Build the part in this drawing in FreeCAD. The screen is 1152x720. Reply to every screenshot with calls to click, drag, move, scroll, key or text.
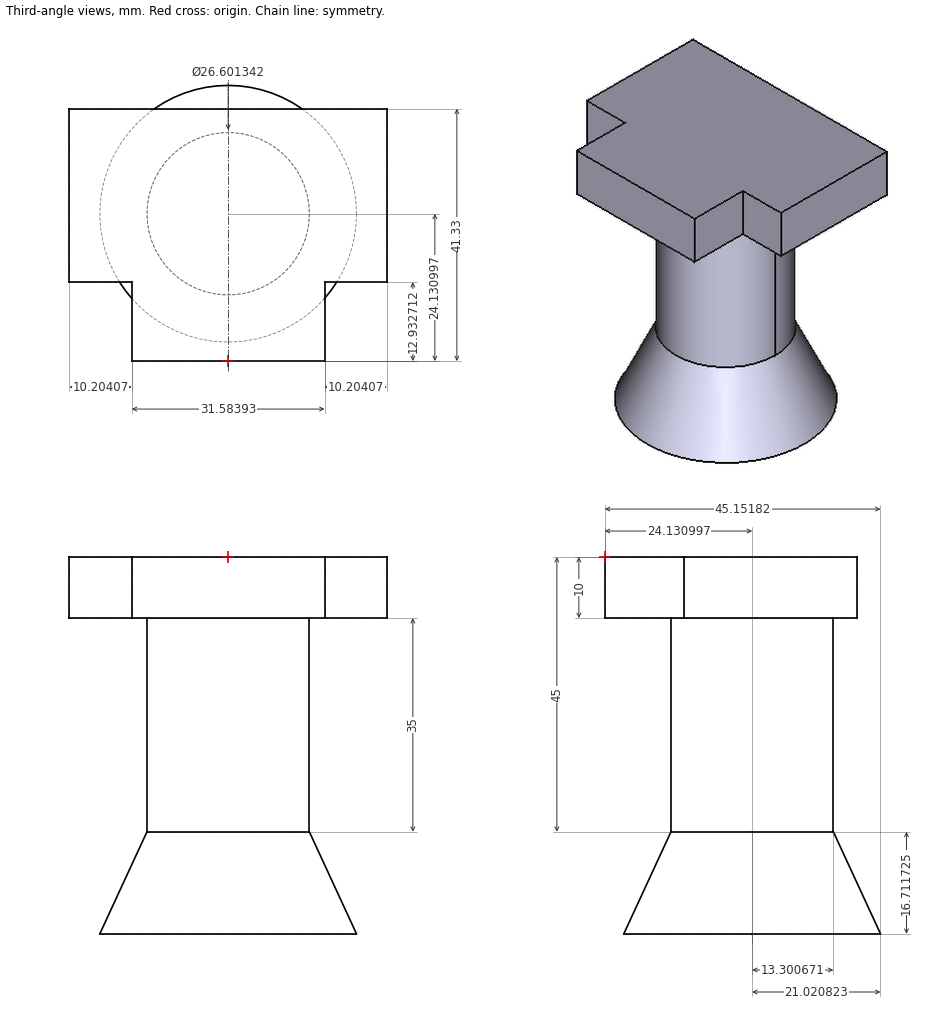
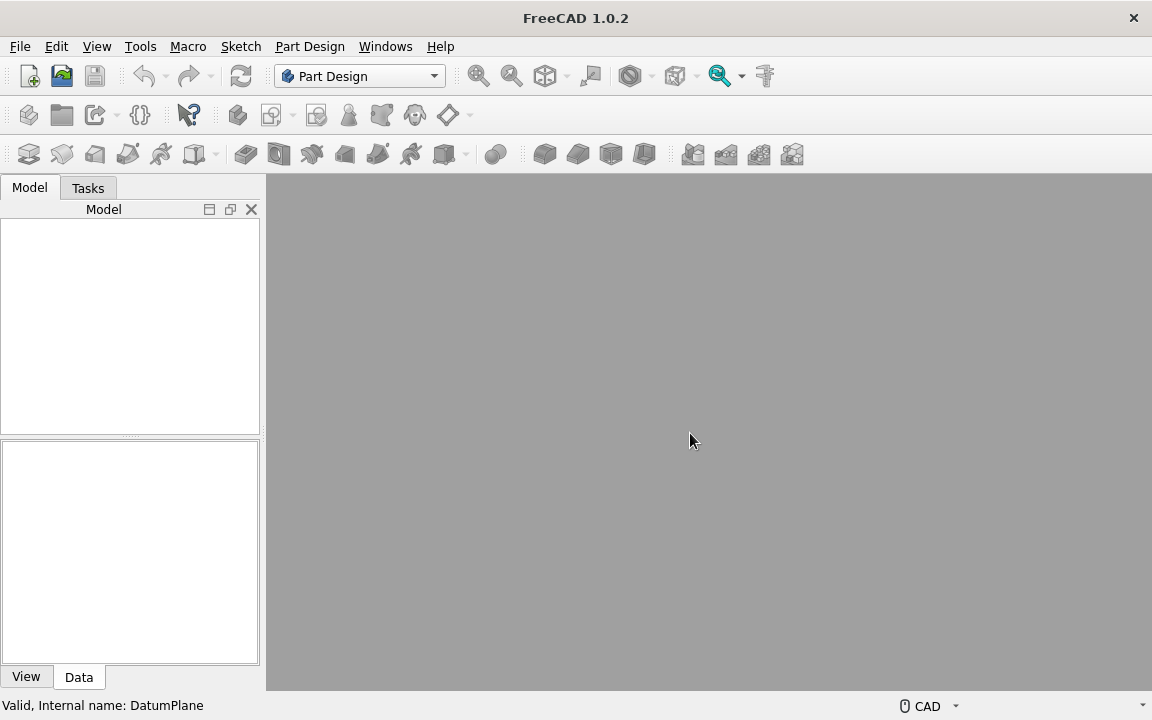
key(ctrl+n)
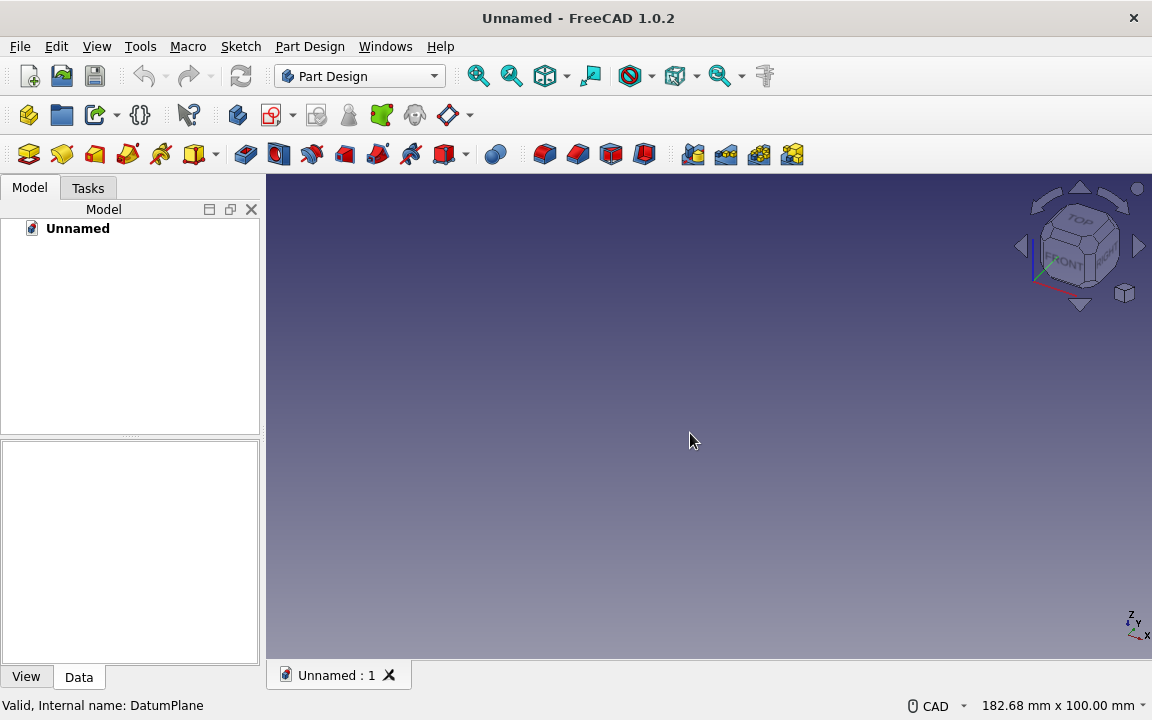
click(270, 116)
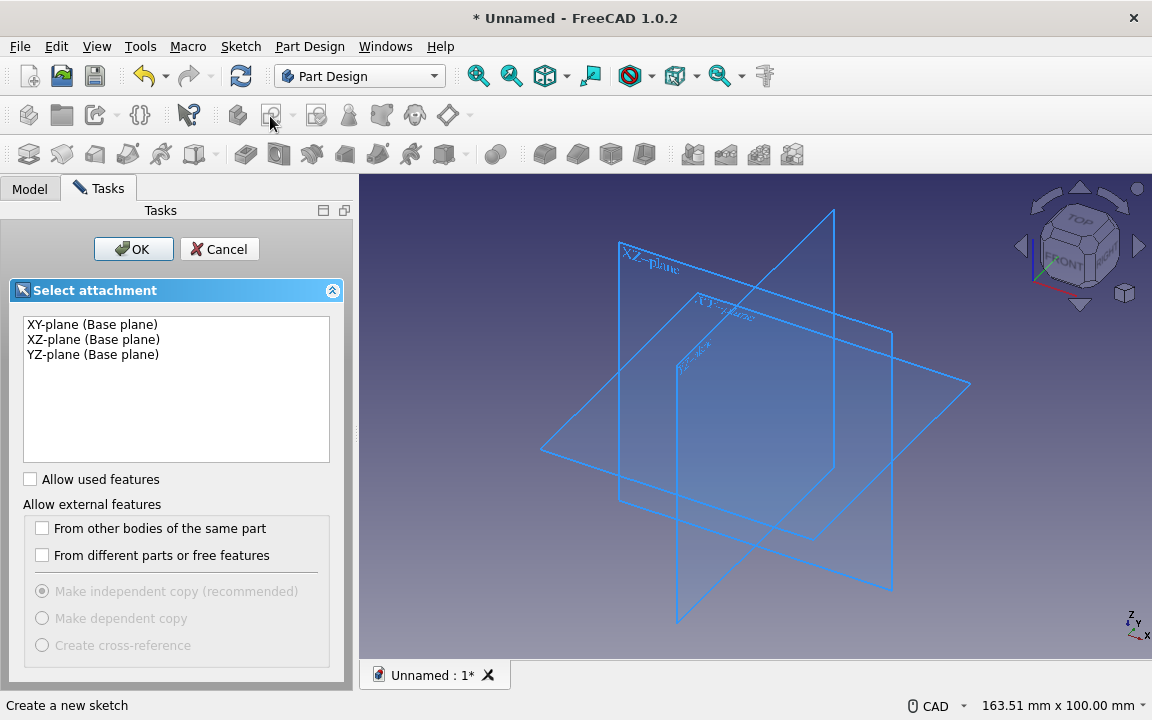
click(84, 324)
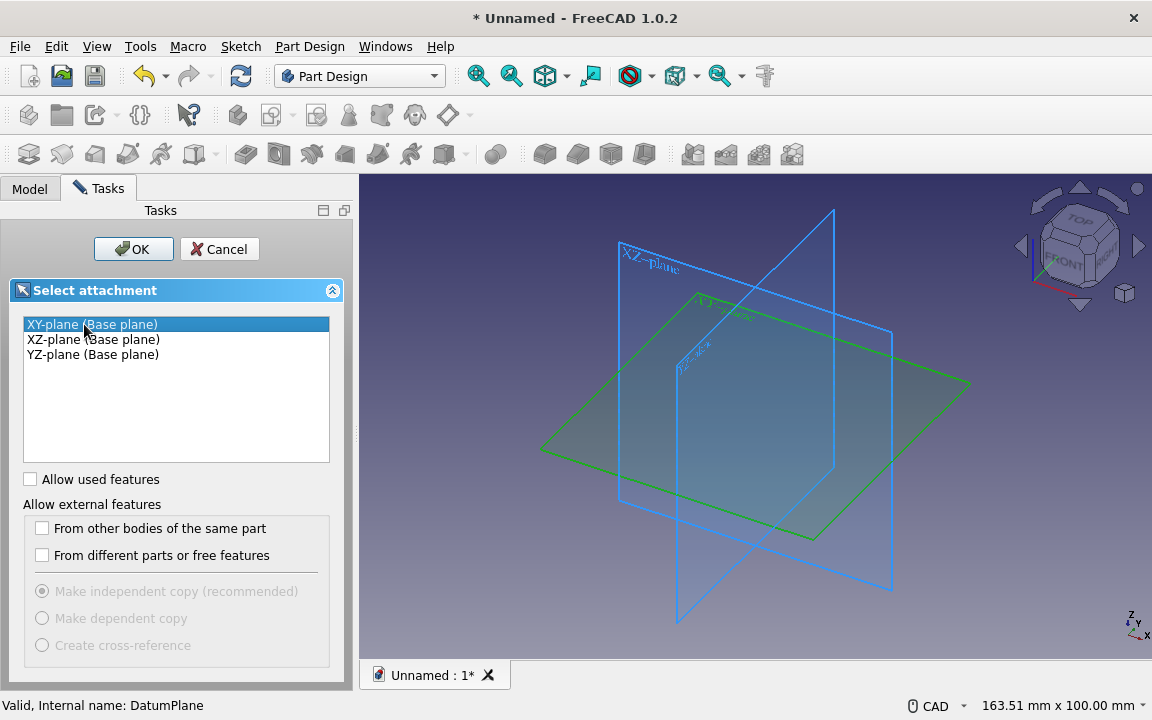
click(134, 249)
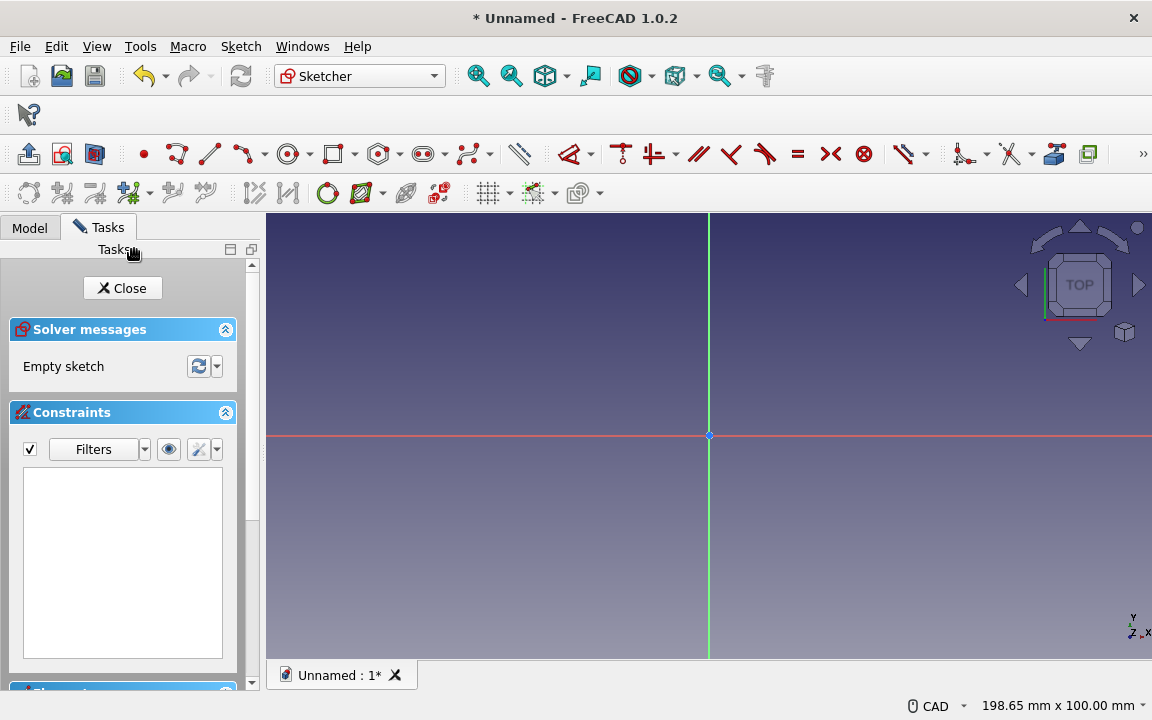
scroll(331, 631, down, 1)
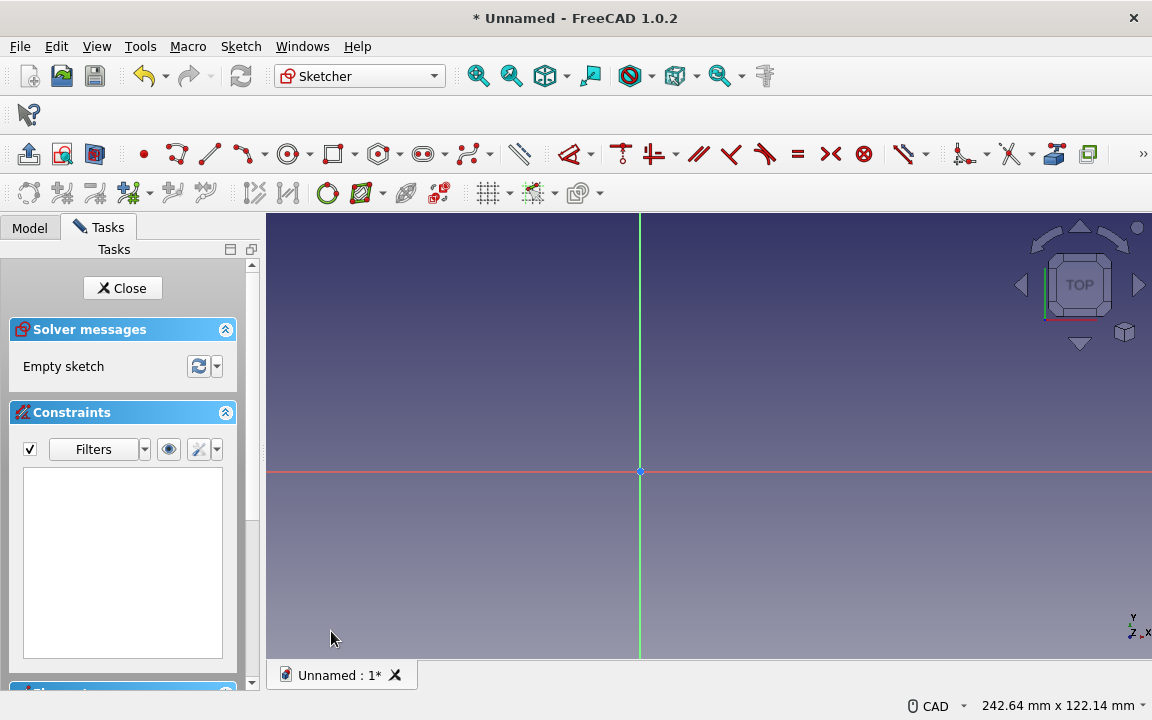
scroll(640, 347, up, 3)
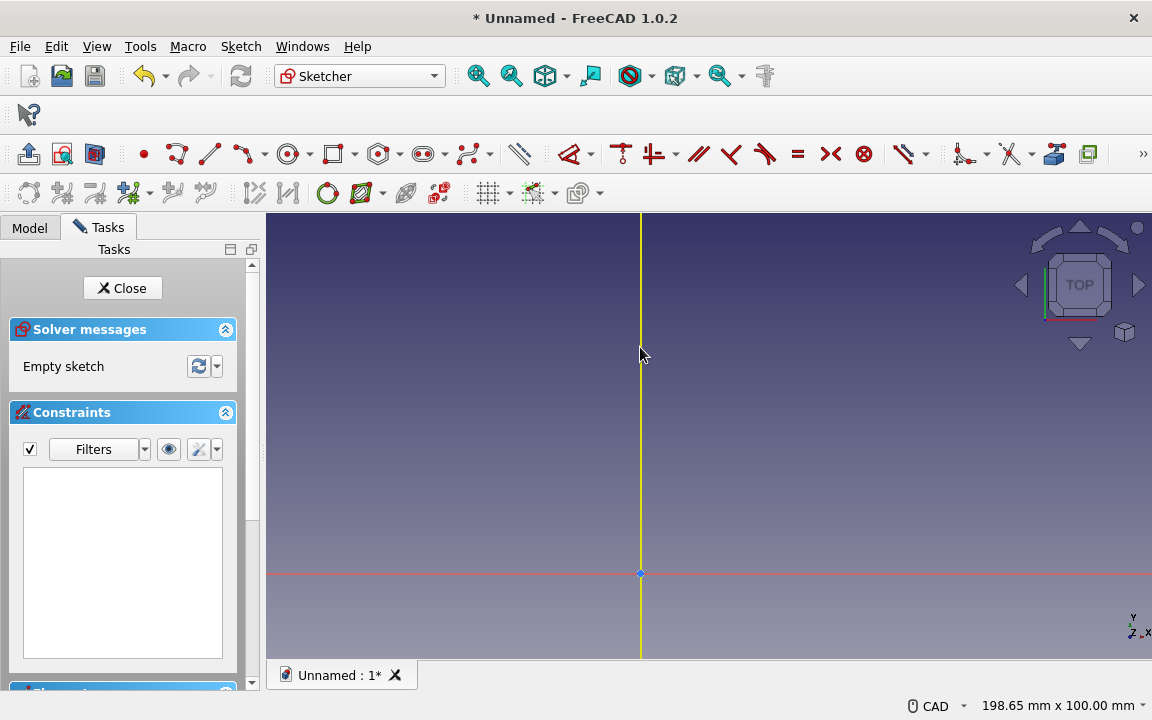
click(177, 154)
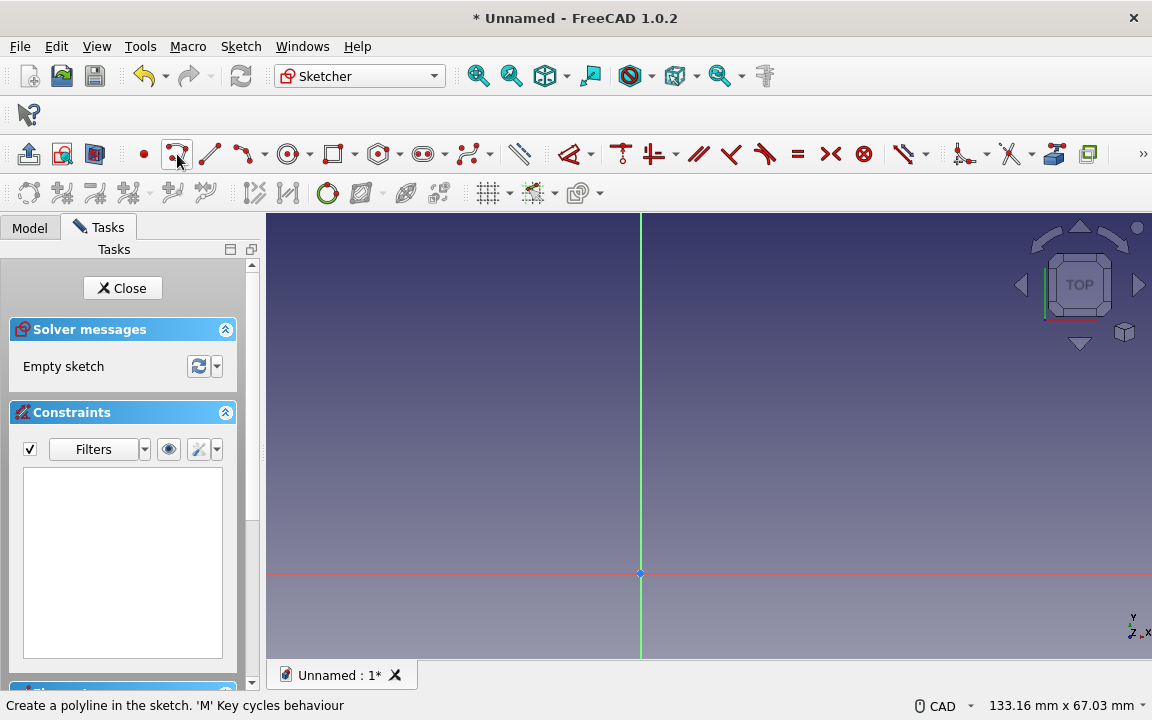
click(535, 574)
click(746, 565)
click(746, 488)
click(814, 488)
click(814, 299)
click(468, 299)
click(468, 488)
click(535, 488)
click(535, 574)
key(Escape)
key(Escape)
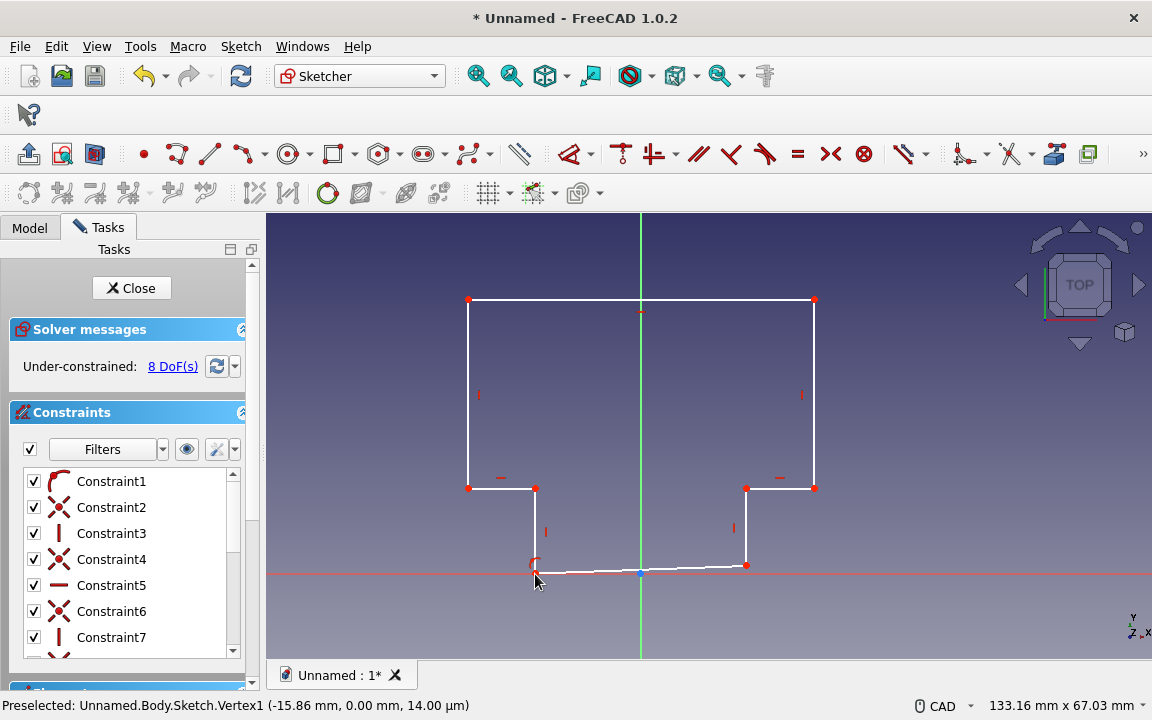
click(598, 571)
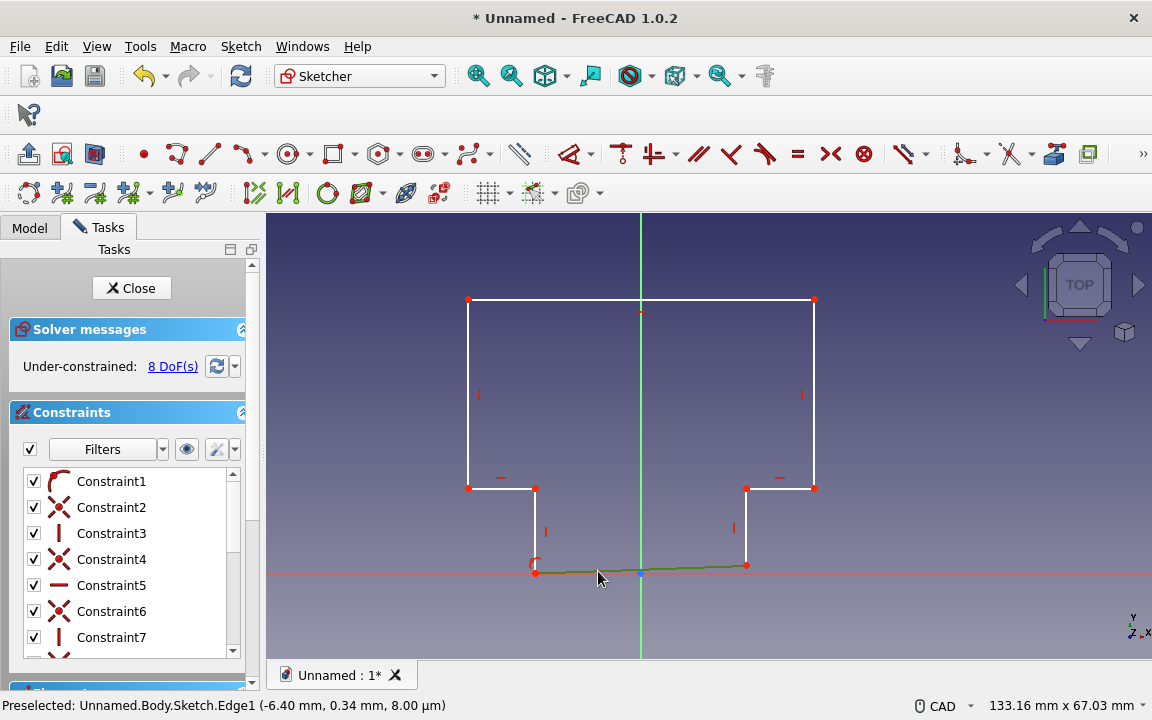
key(h)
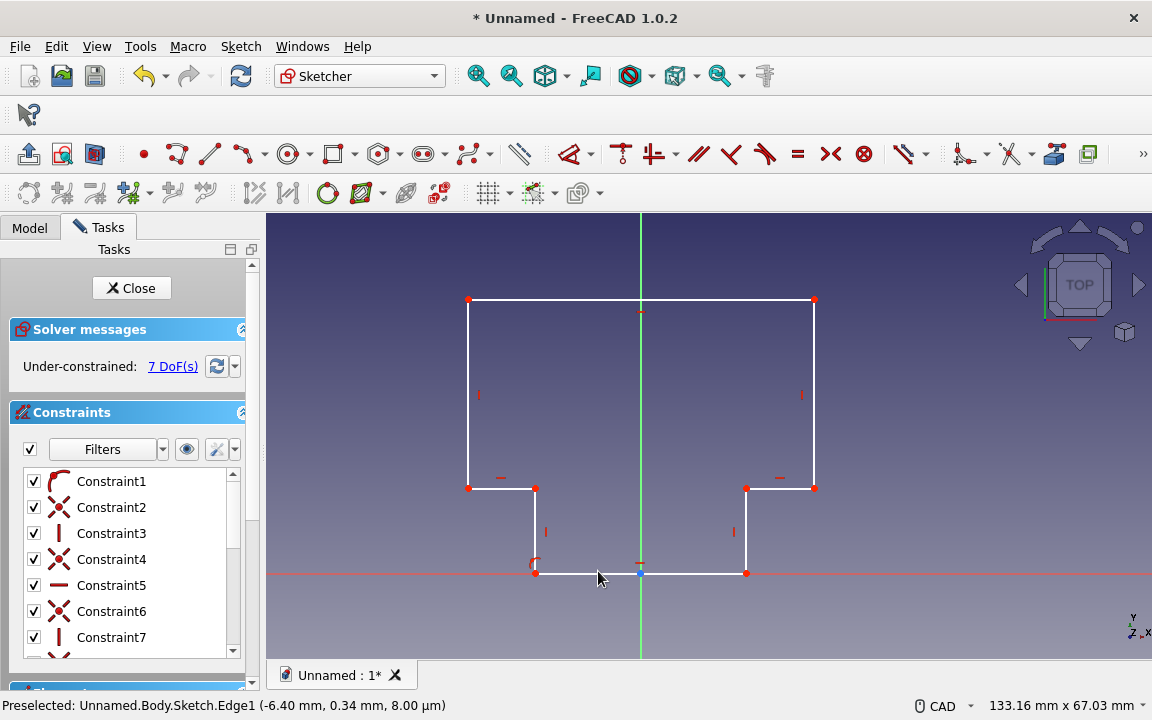
click(814, 489)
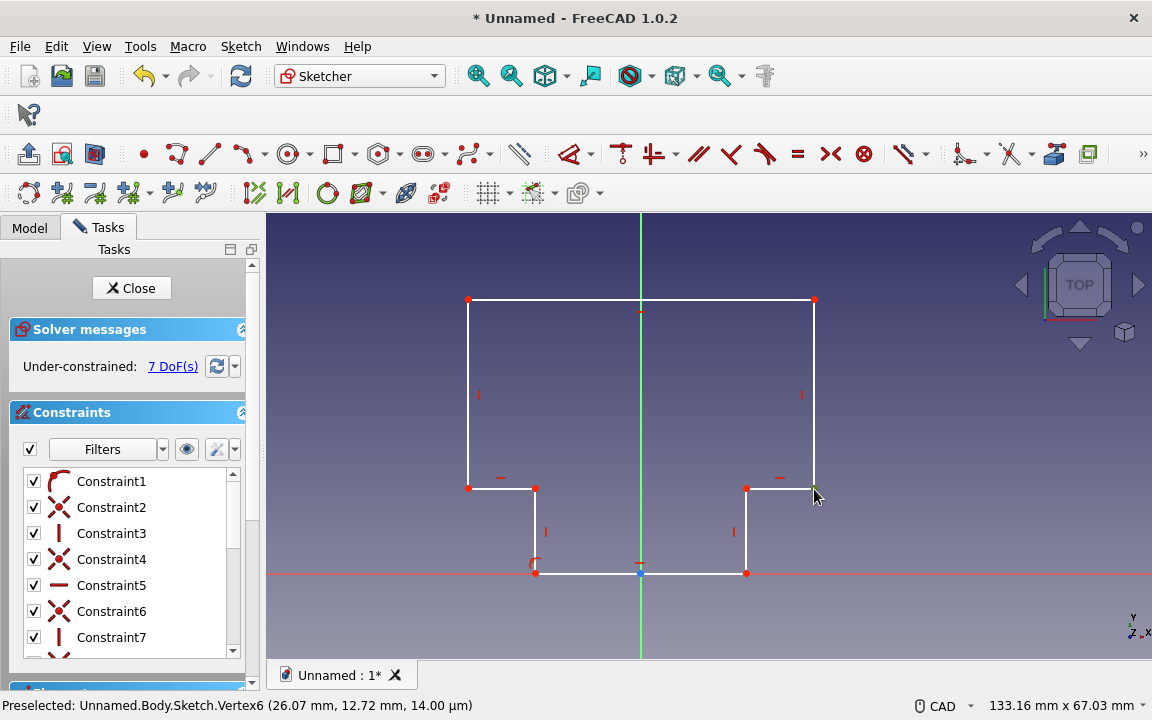
click(468, 489)